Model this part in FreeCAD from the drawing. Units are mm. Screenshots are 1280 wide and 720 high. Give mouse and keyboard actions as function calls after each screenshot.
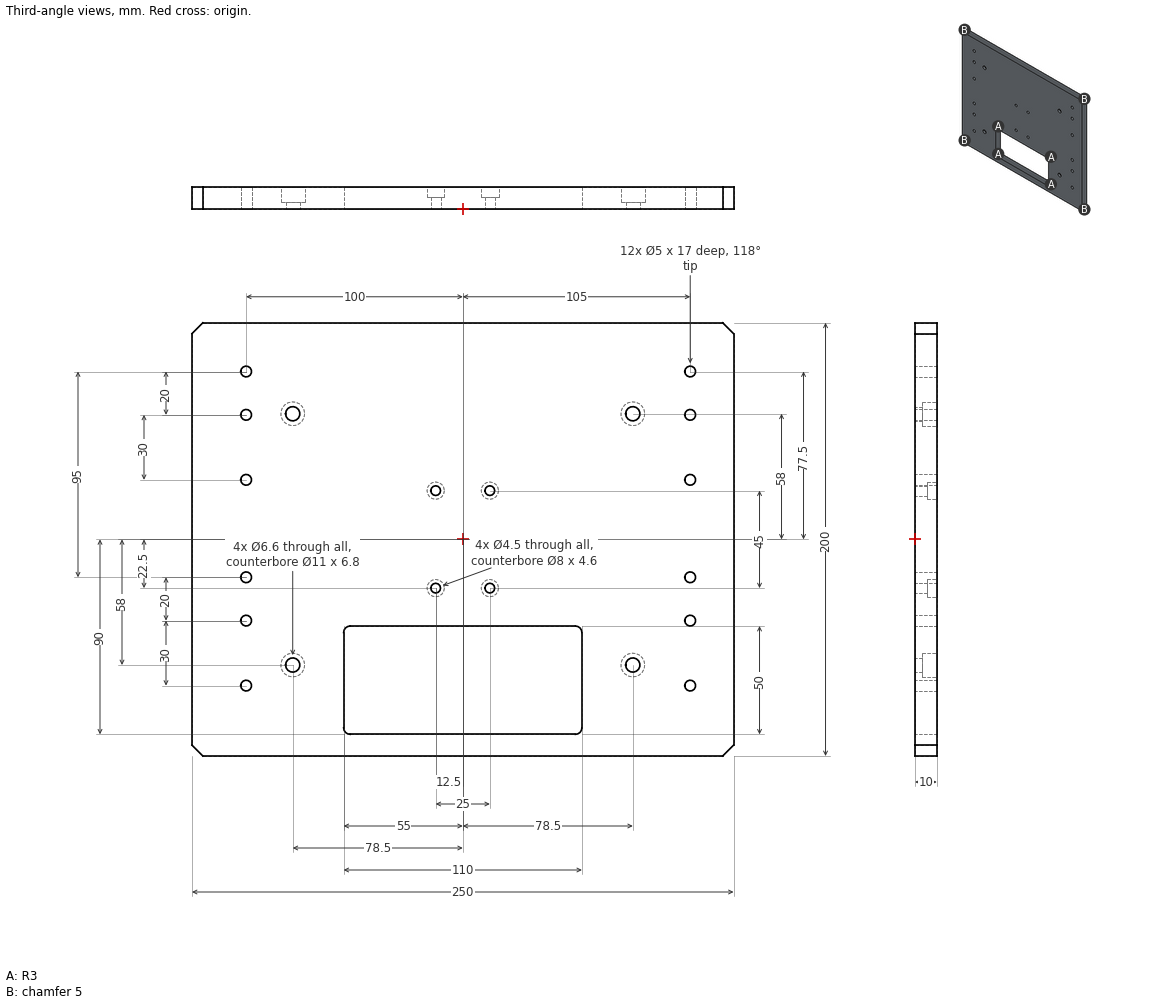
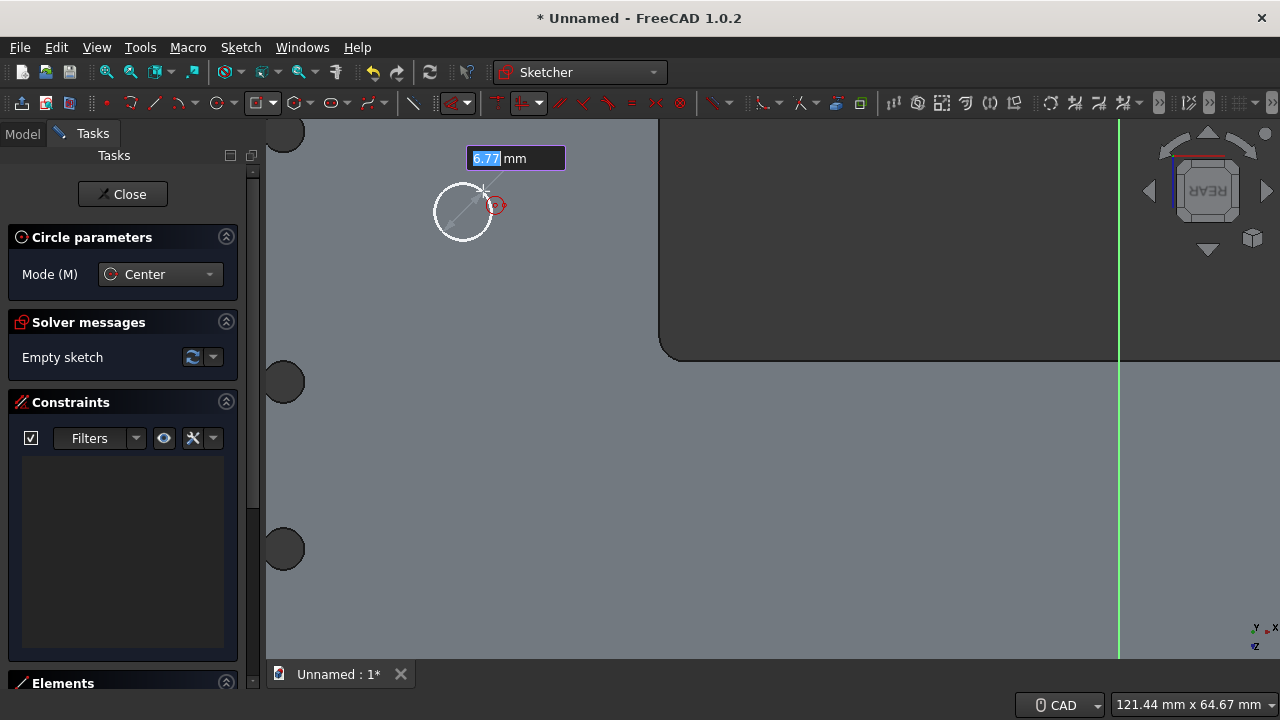
text(6.6)
key(Return)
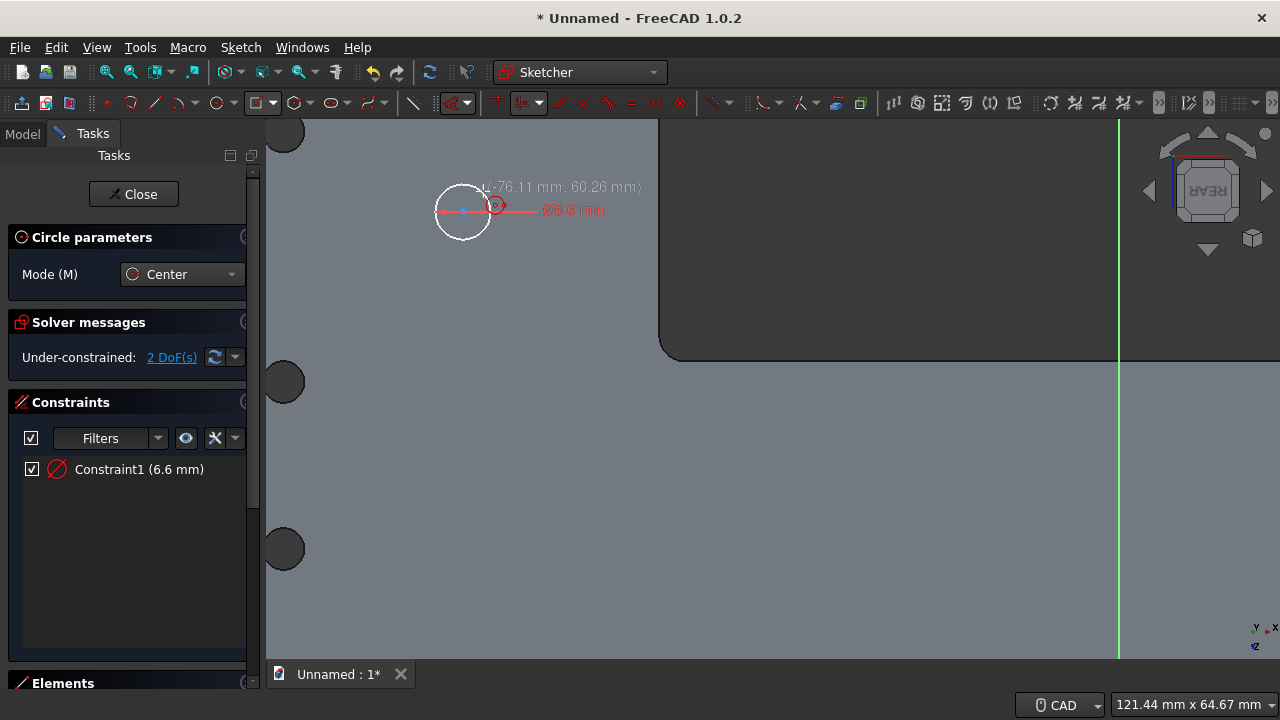
scroll(464, 211, down, 5)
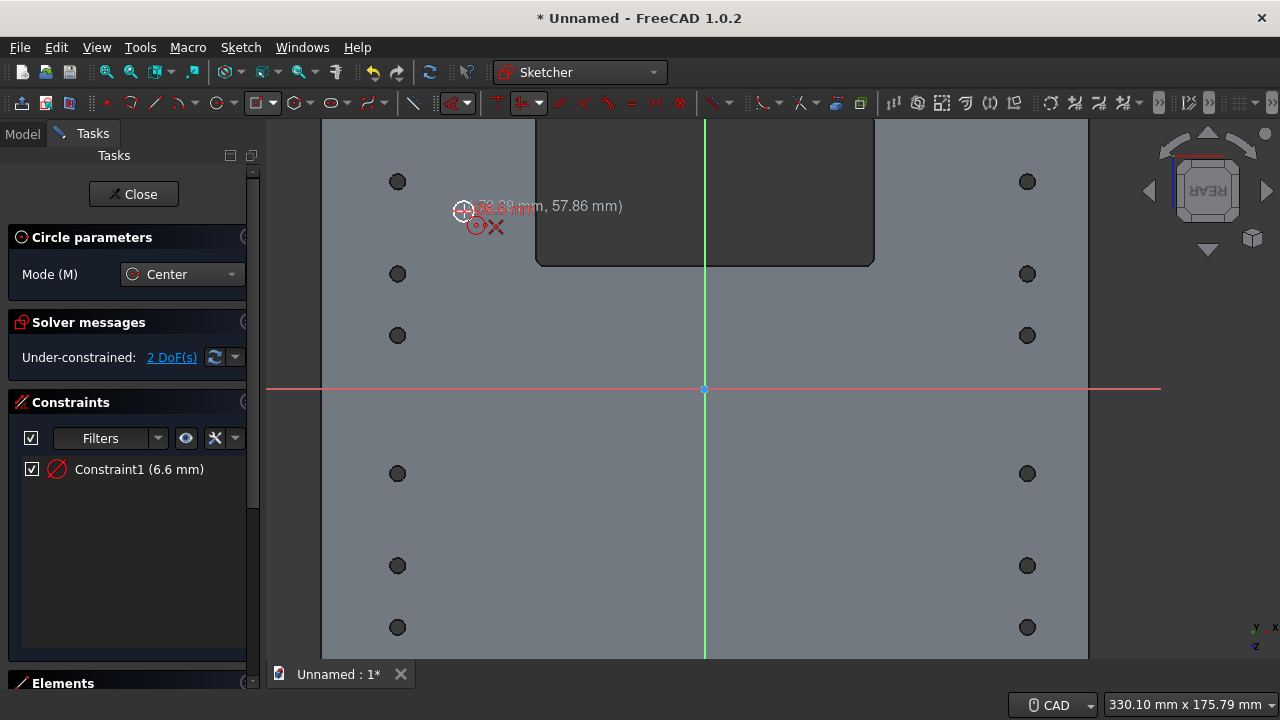
scroll(946, 211, up, 5)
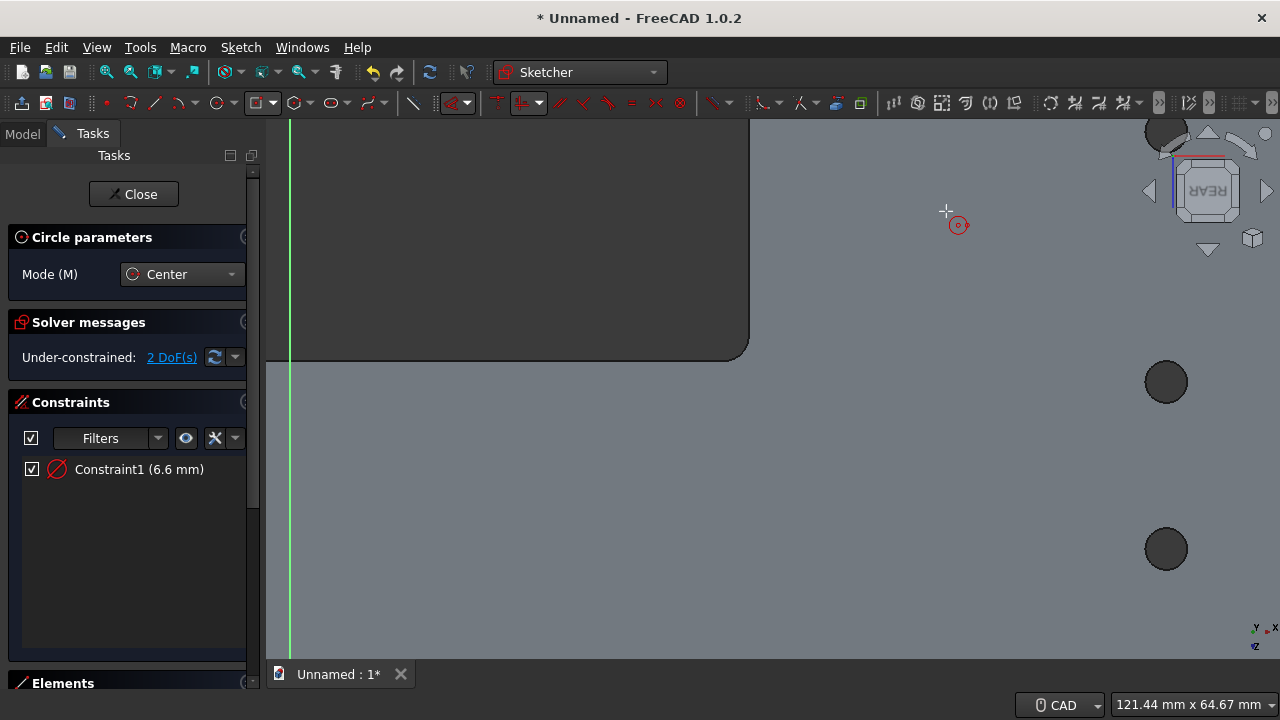
click(945, 211)
move(964, 191)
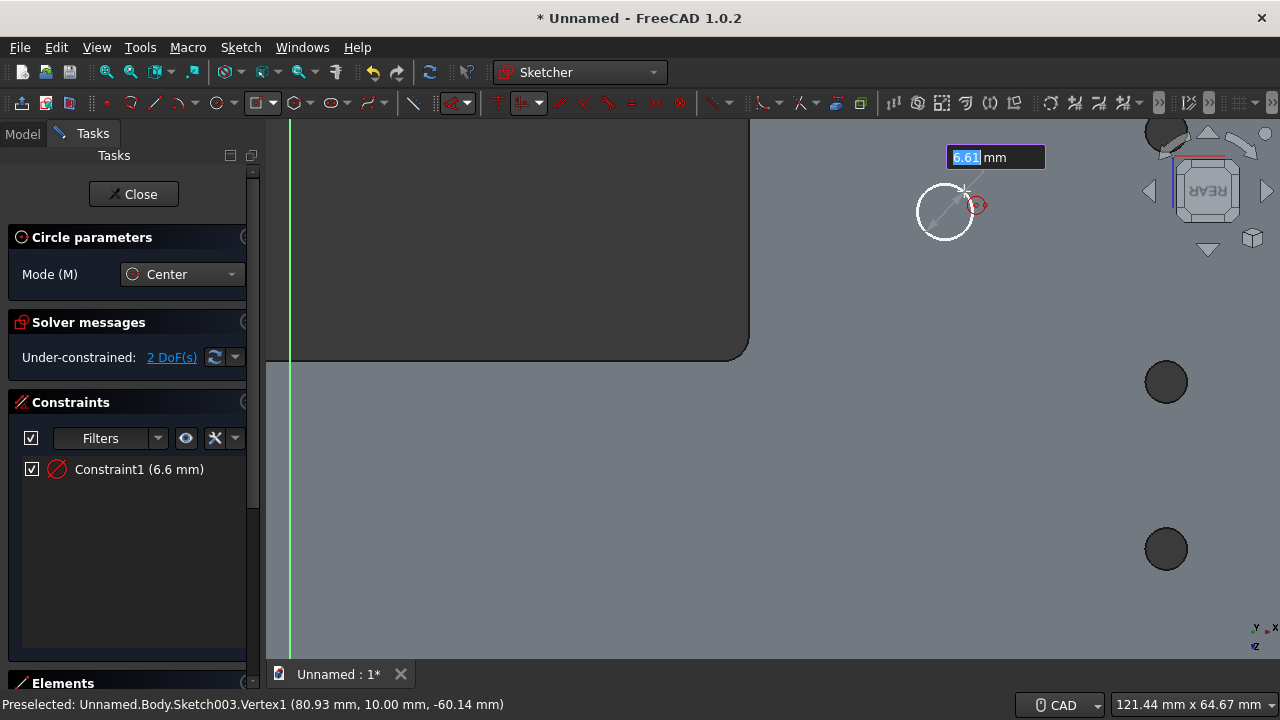
text(6.6)
key(Return)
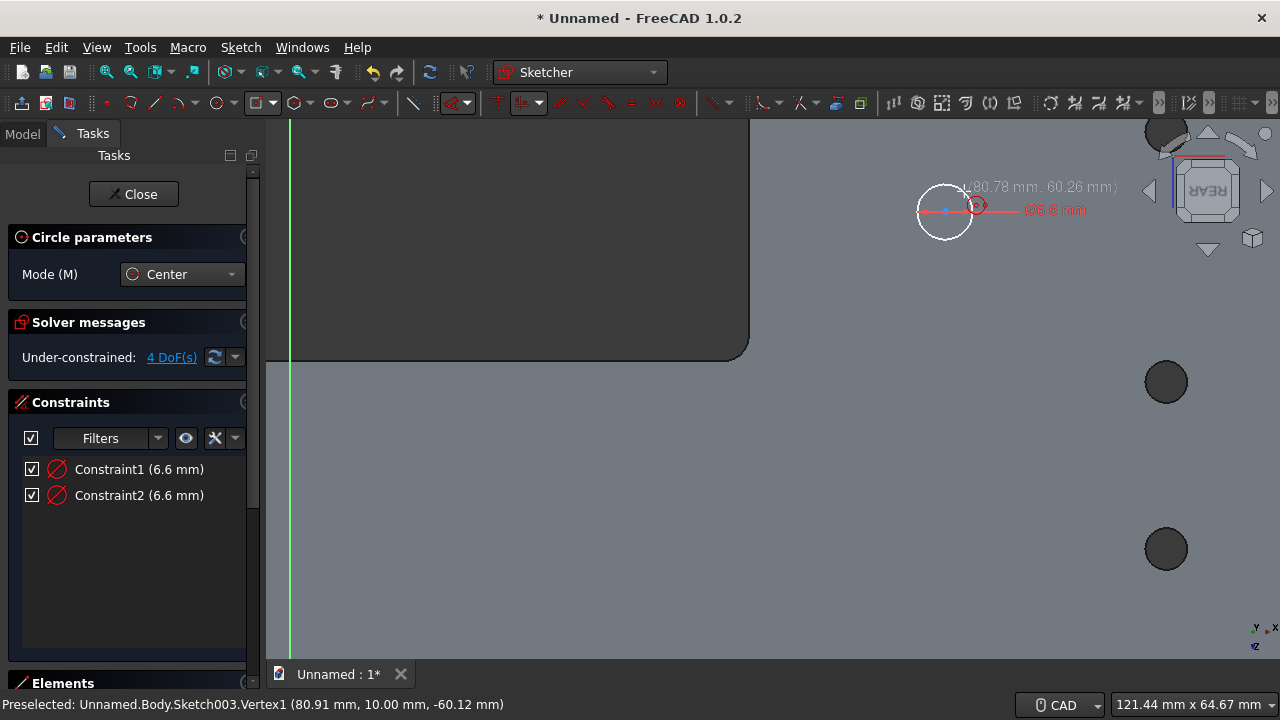
scroll(946, 211, down, 5)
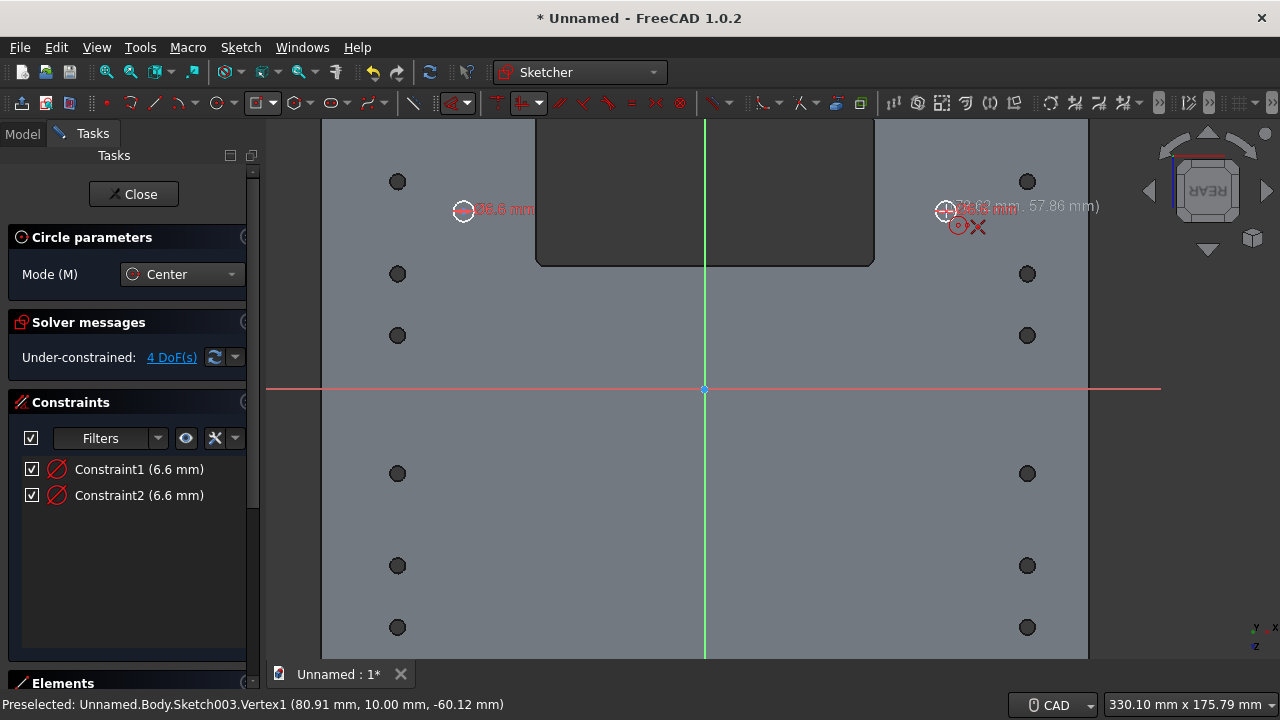
scroll(946, 567, up, 5)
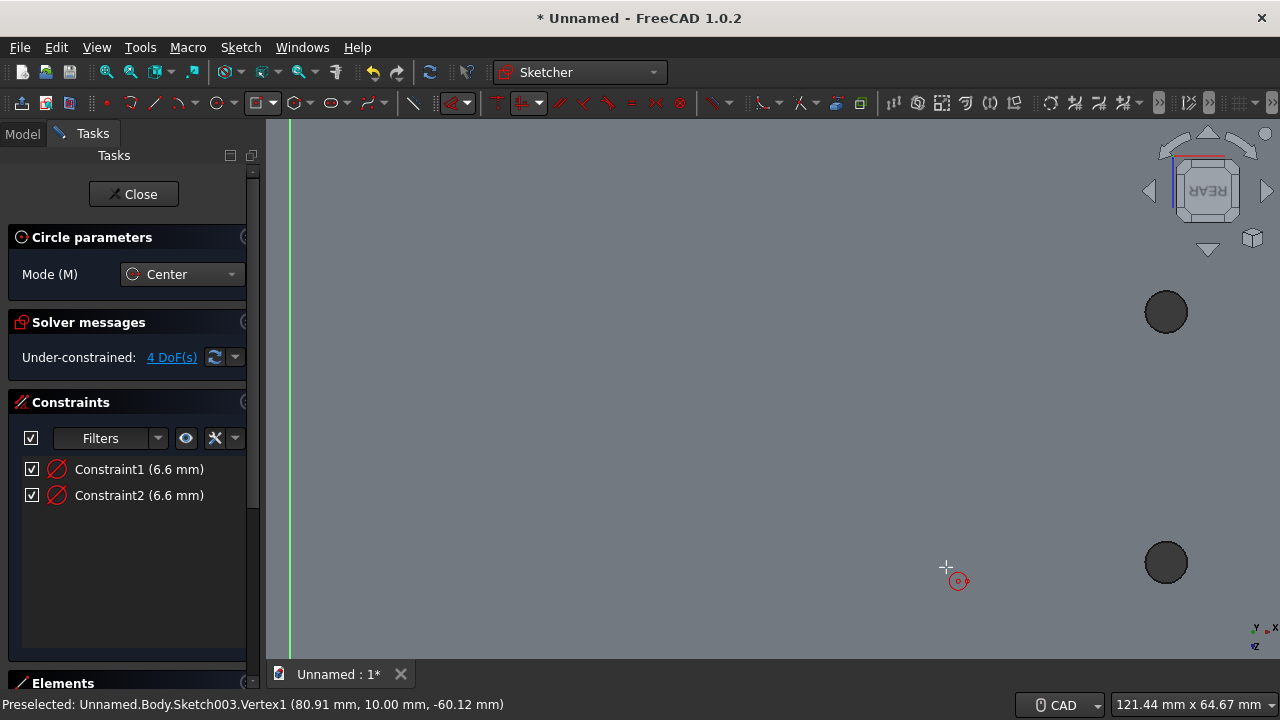
click(945, 567)
move(964, 547)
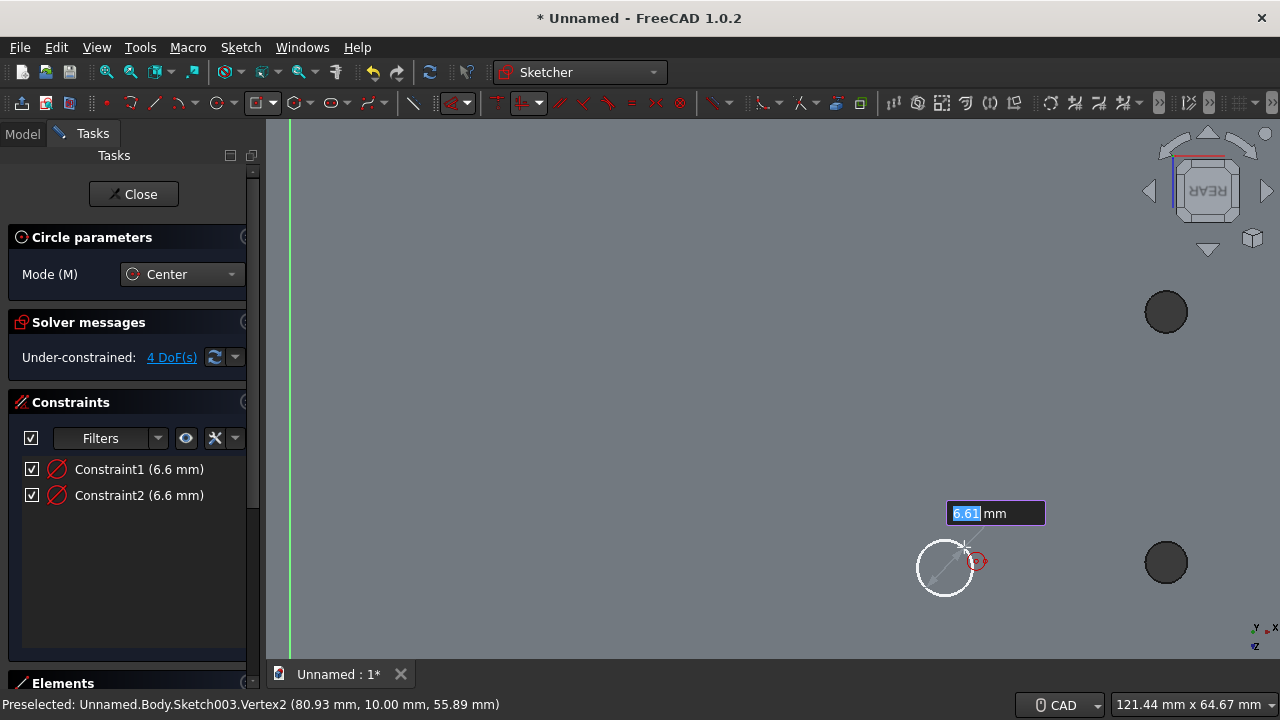
text(6.6)
key(Return)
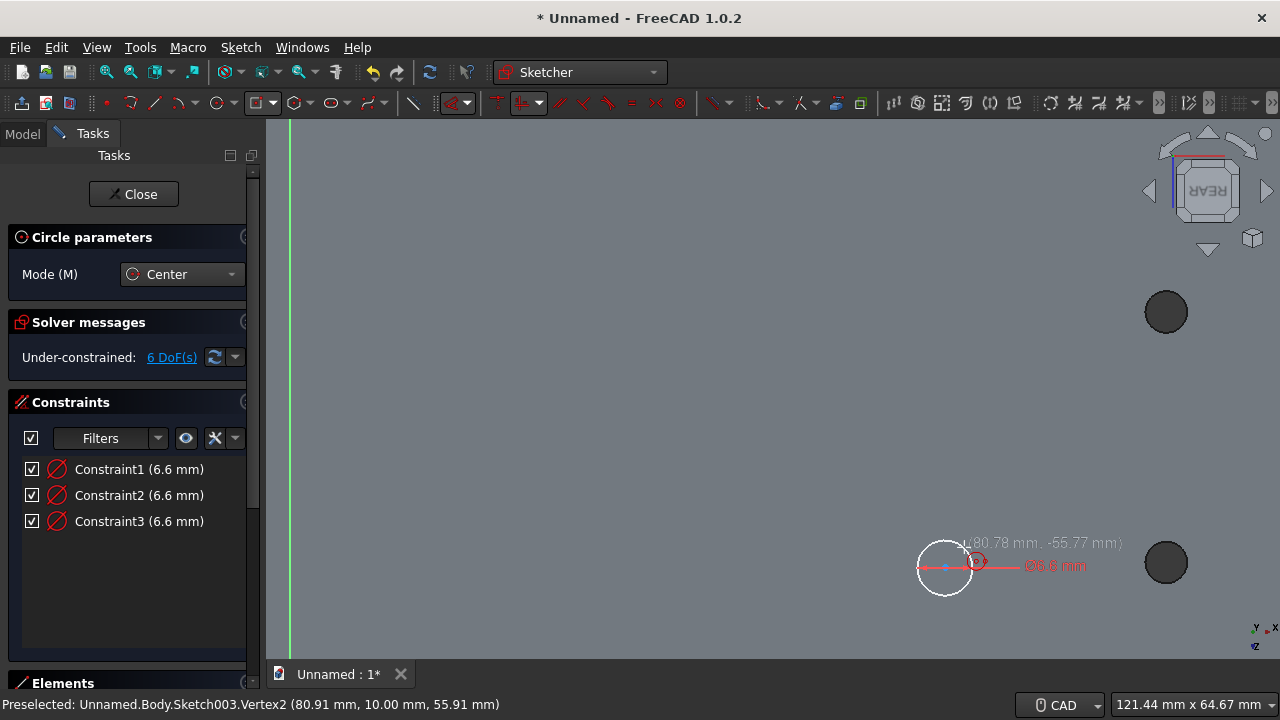
scroll(946, 567, down, 5)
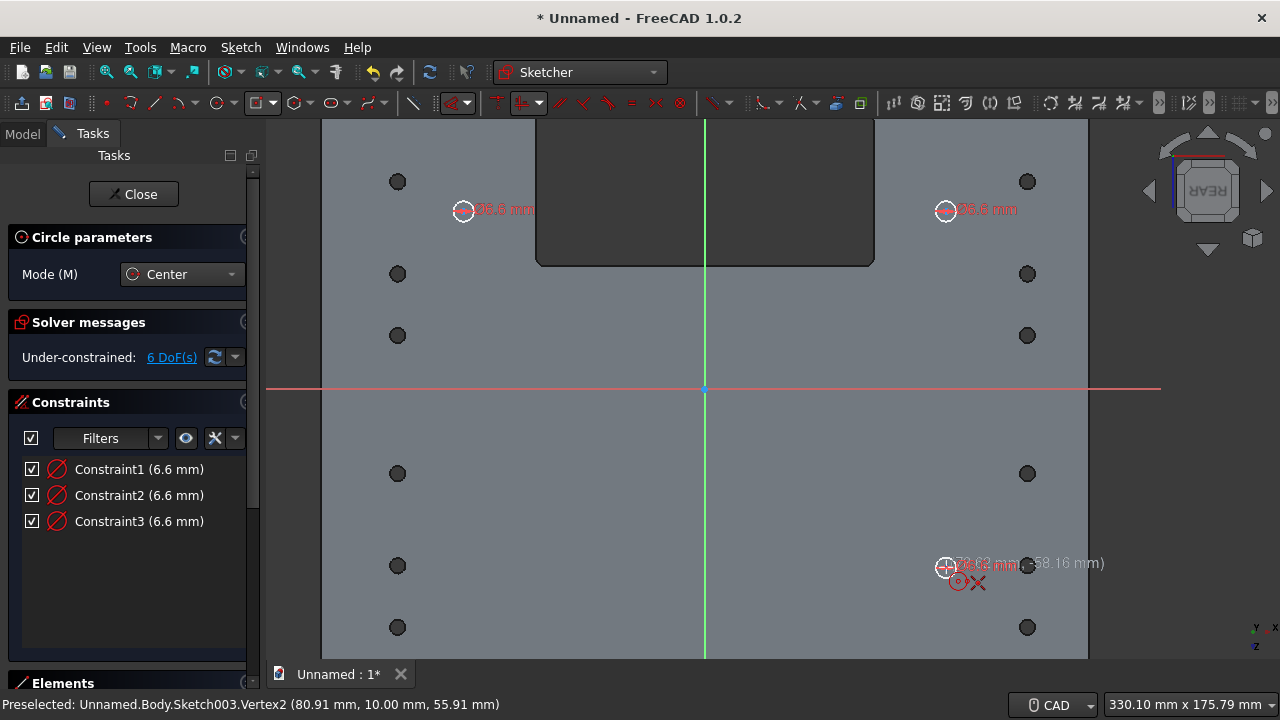
scroll(464, 567, up, 5)